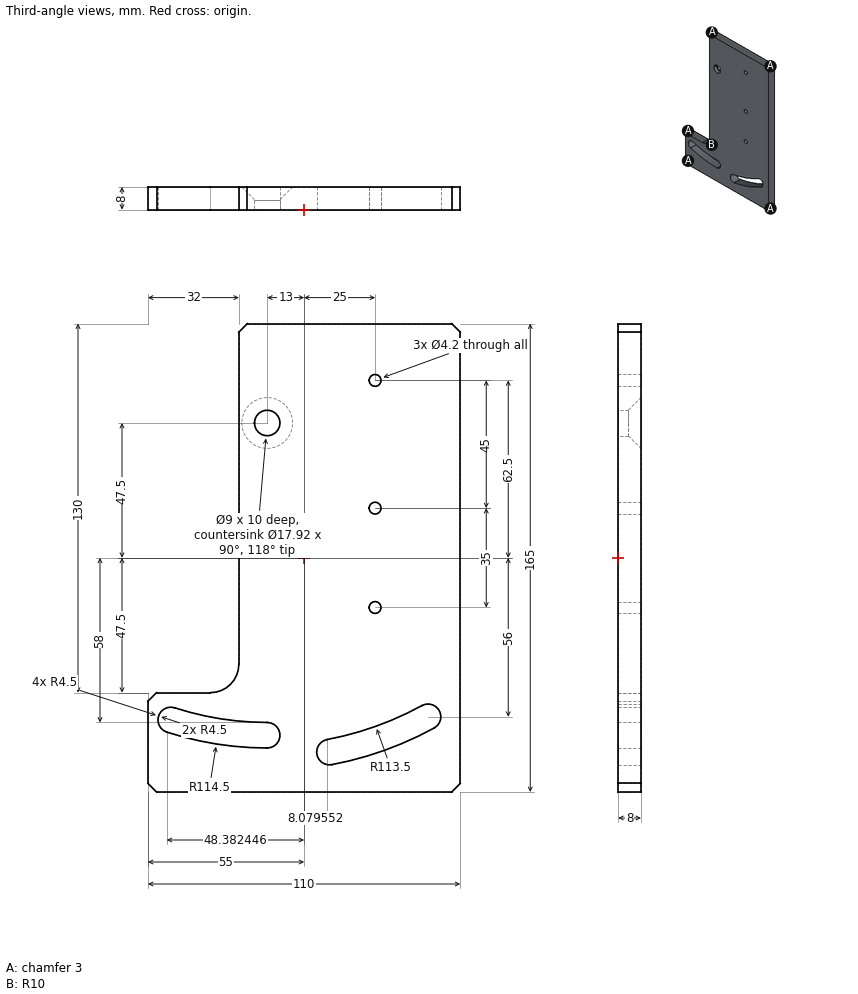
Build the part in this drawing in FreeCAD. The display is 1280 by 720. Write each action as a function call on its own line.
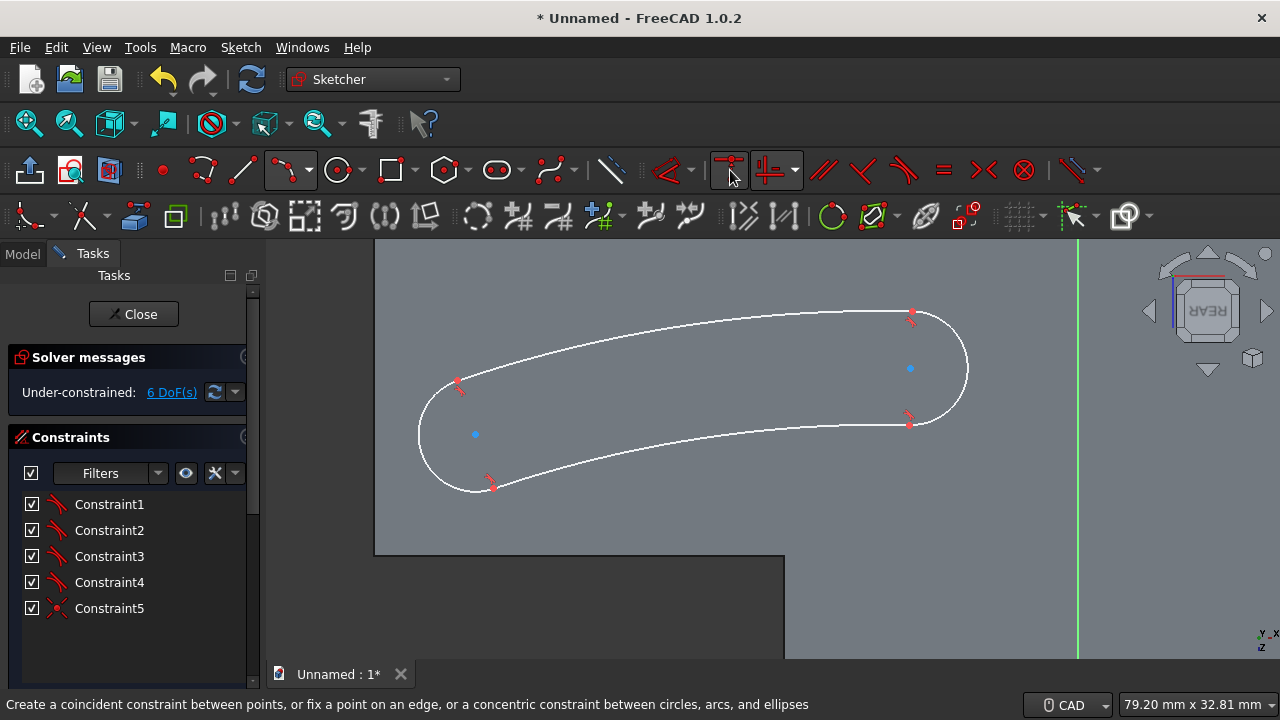
click(666, 170)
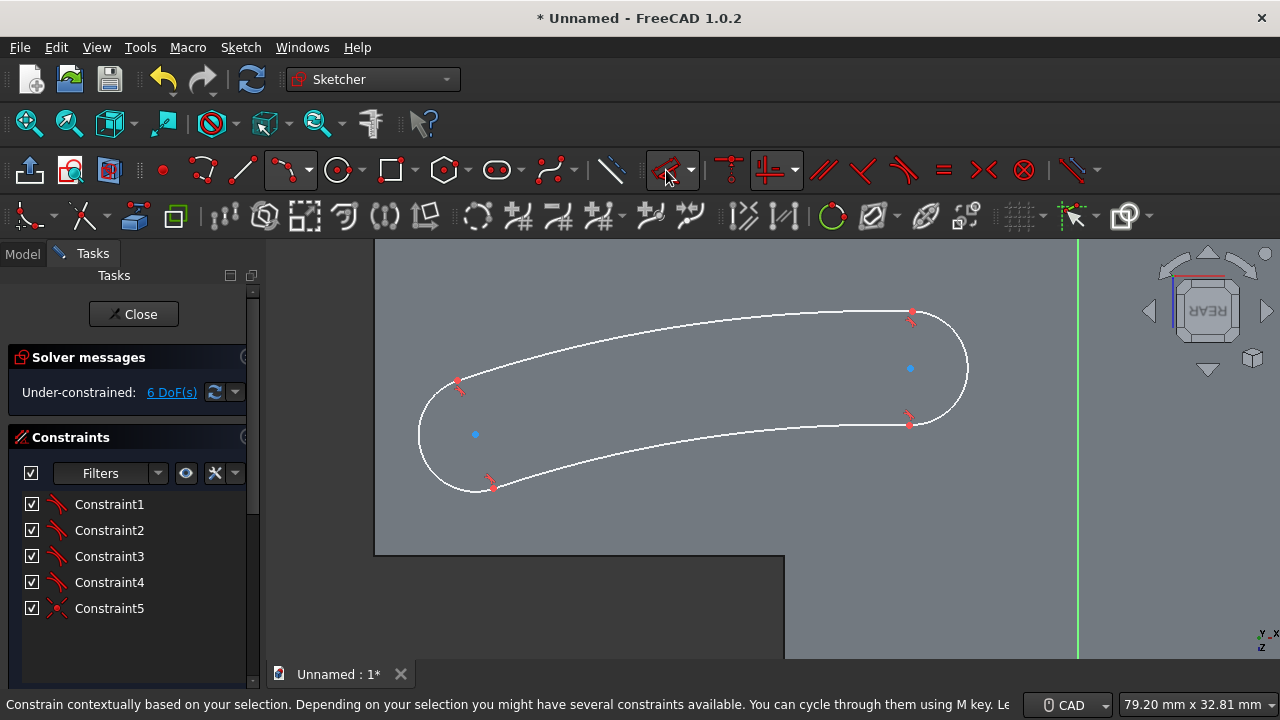
click(956, 403)
click(981, 423)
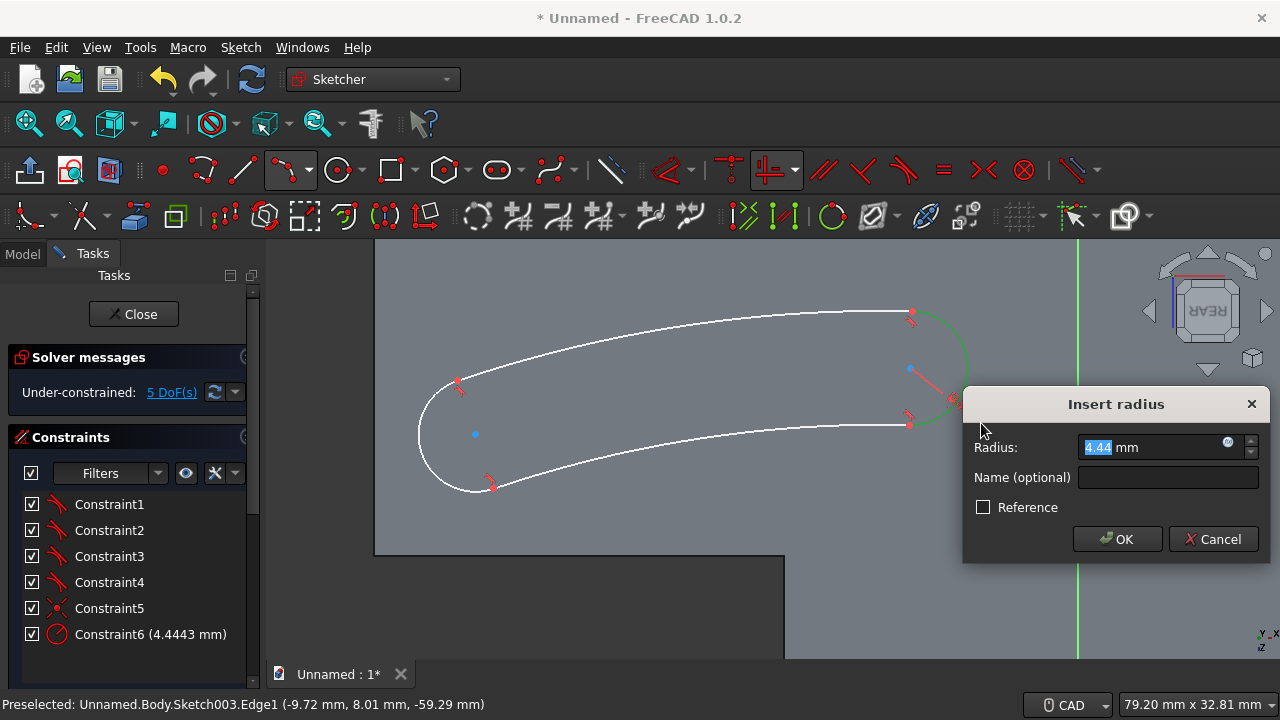
text(4.5)
key(Return)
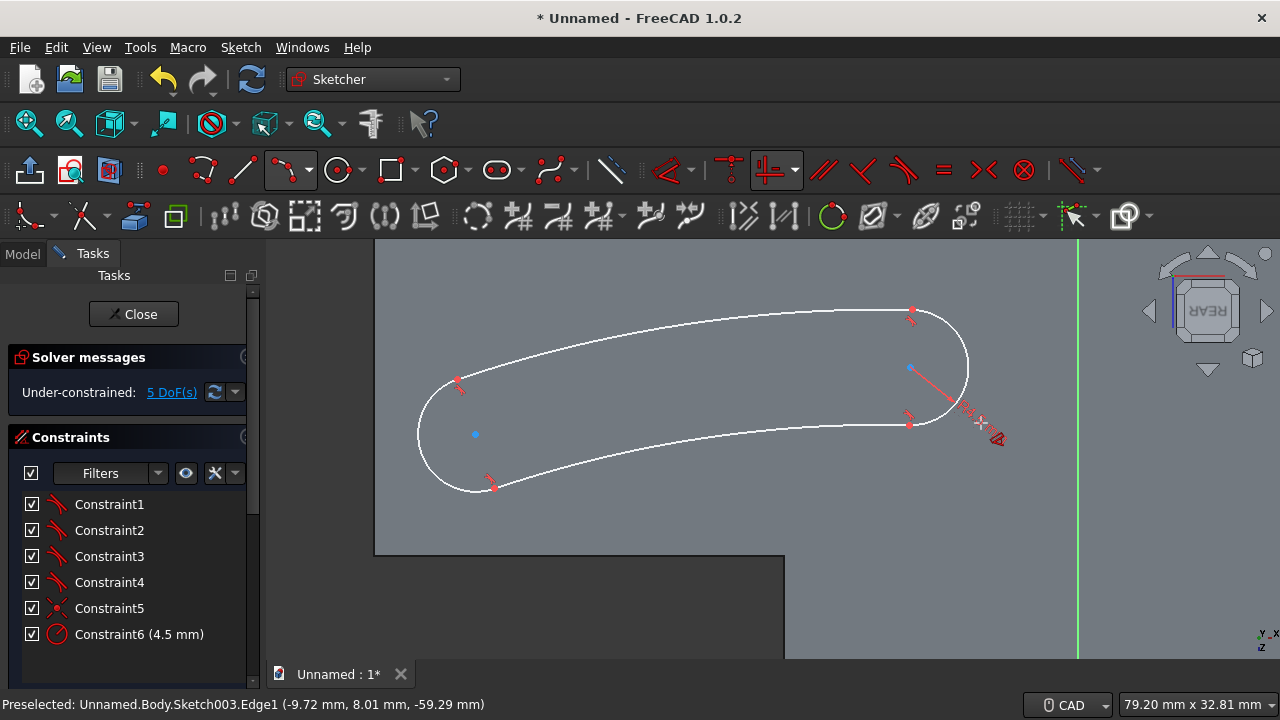
click(774, 314)
click(771, 282)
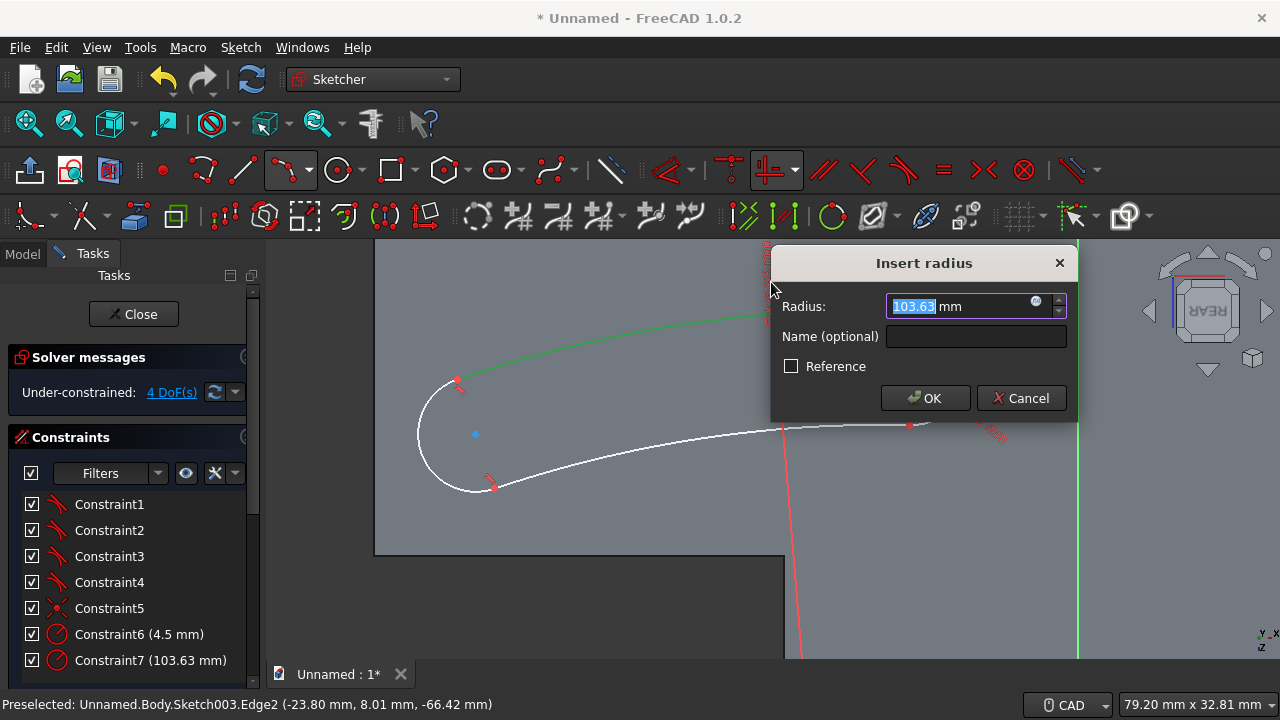
text(114.5)
key(Return)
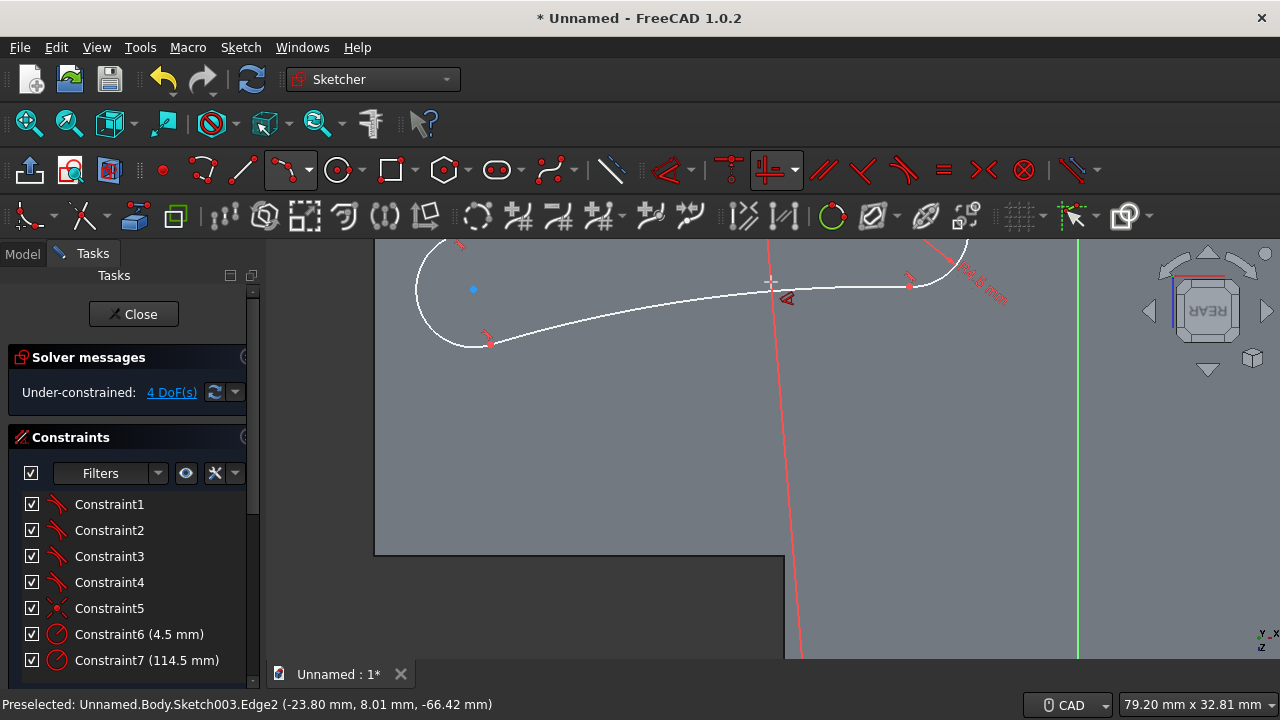
click(910, 287)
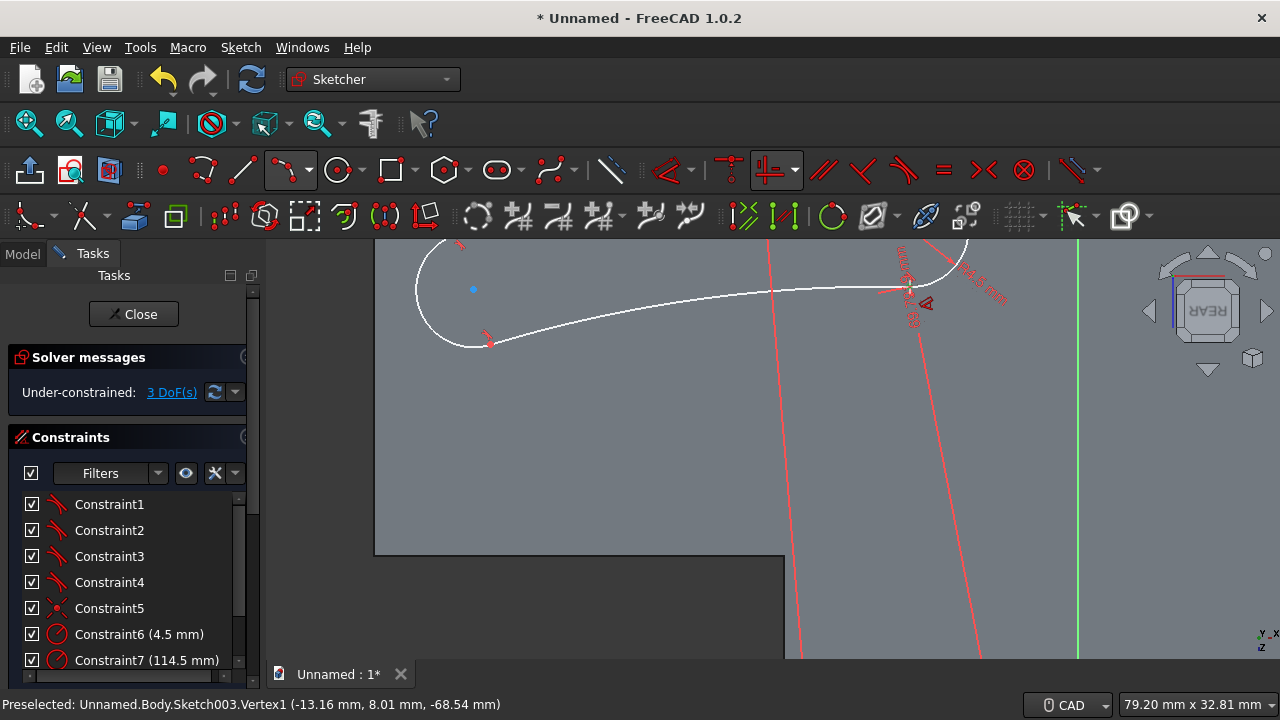
key(Escape)
key(Escape)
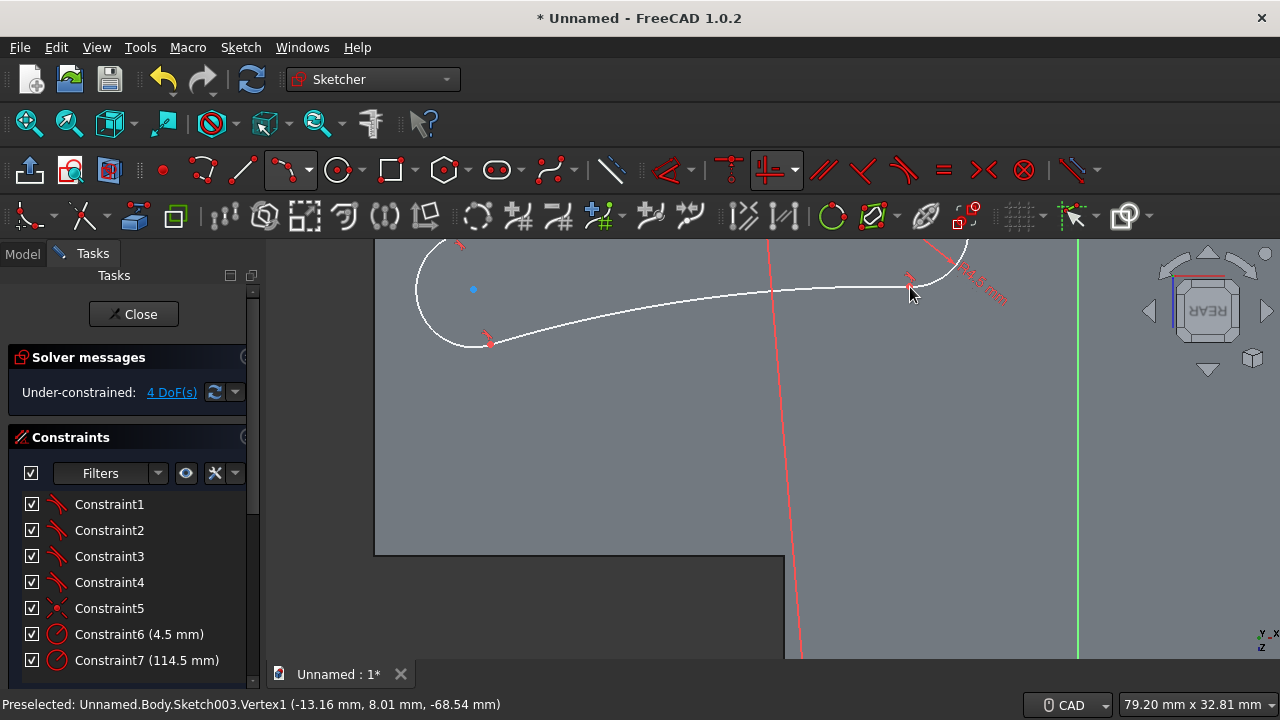
click(910, 287)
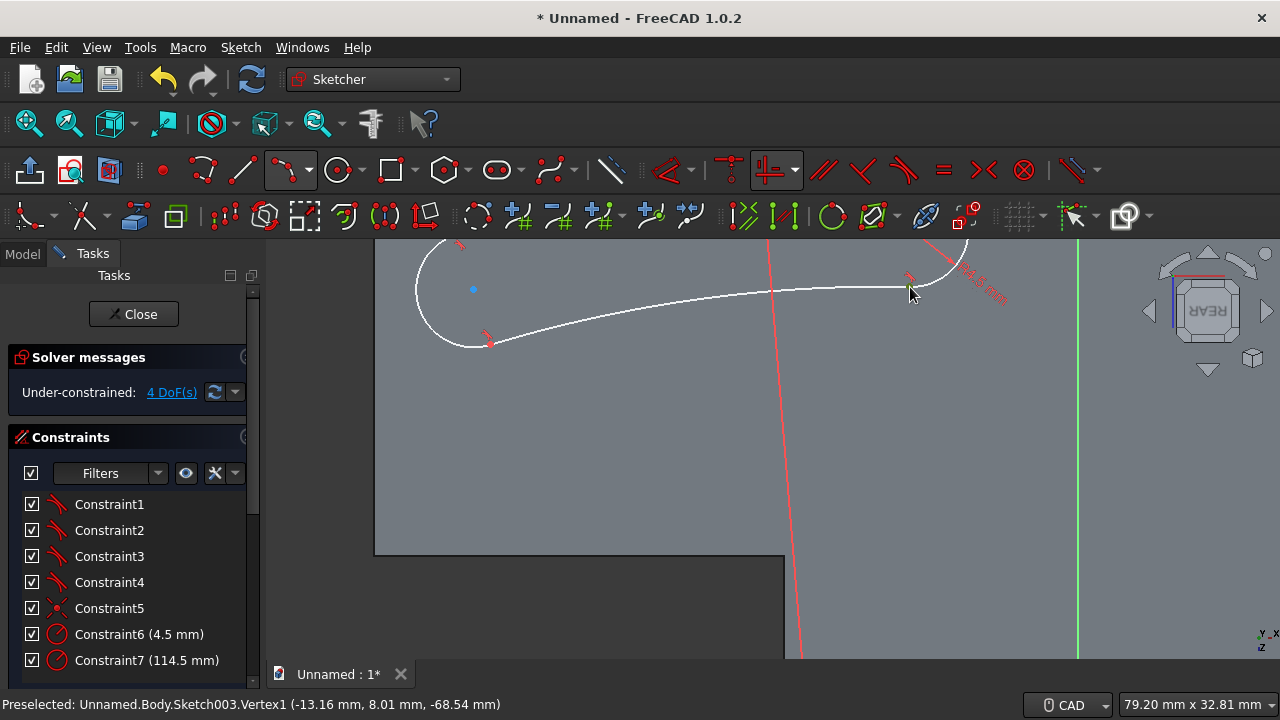
click(694, 170)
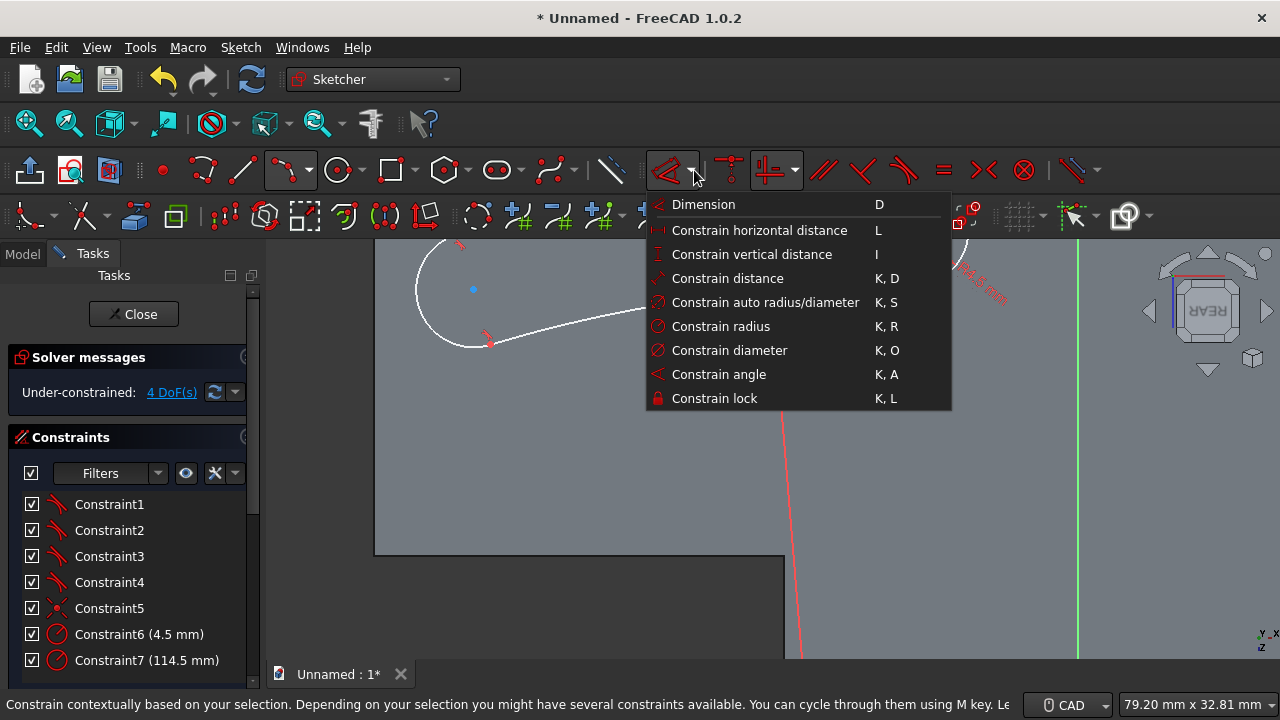
click(799, 230)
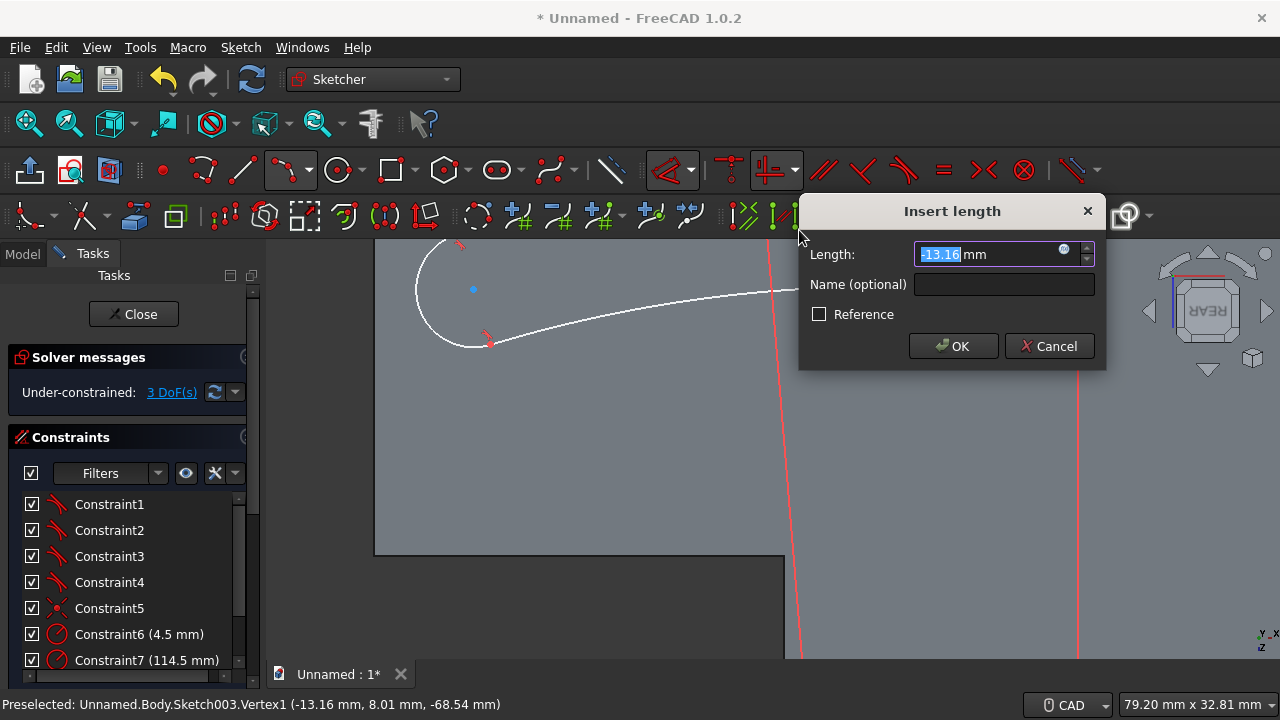
text(-13)
key(Return)